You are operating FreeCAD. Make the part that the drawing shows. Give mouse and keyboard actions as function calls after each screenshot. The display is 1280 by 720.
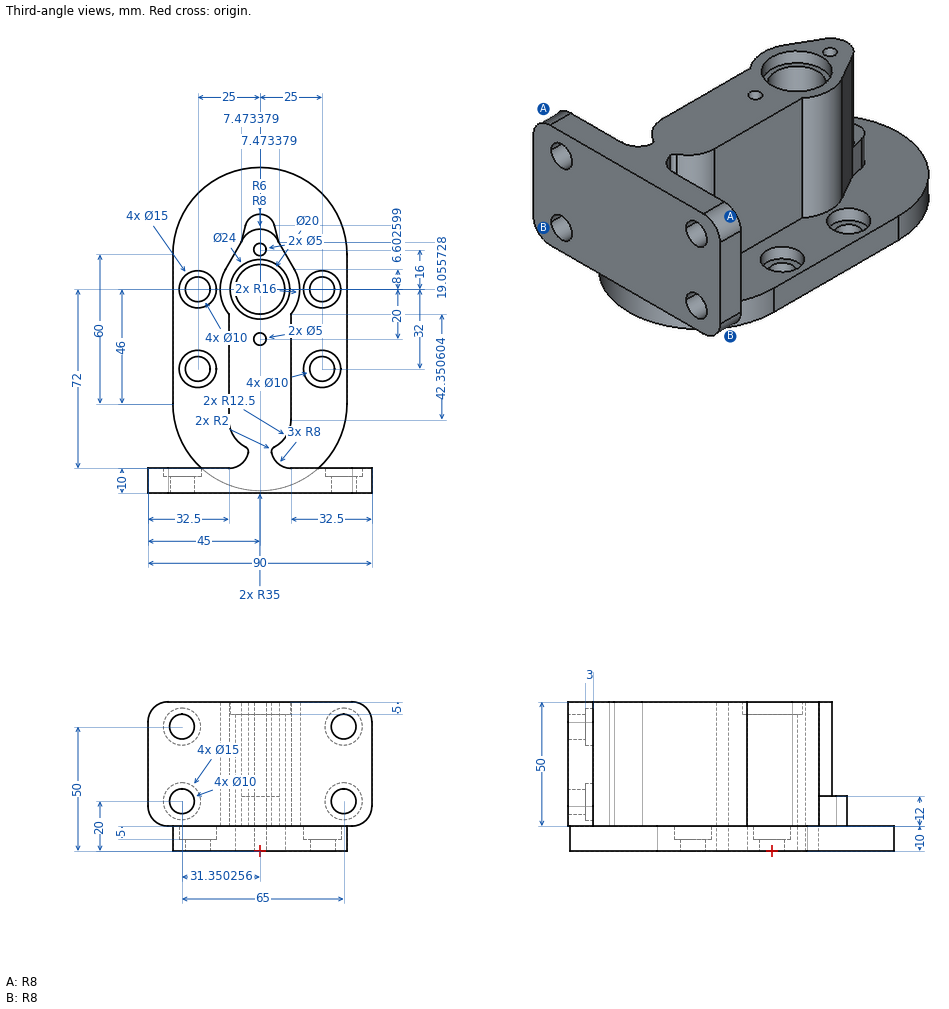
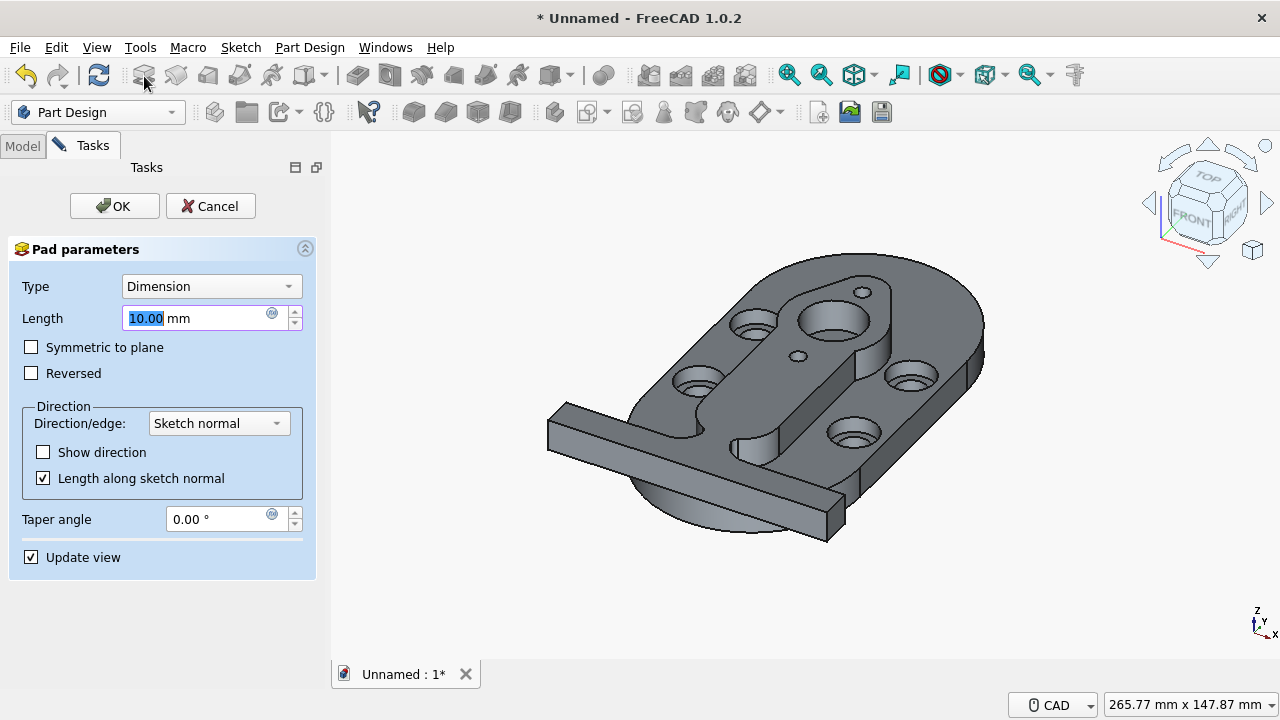
text(50)
key(Tab)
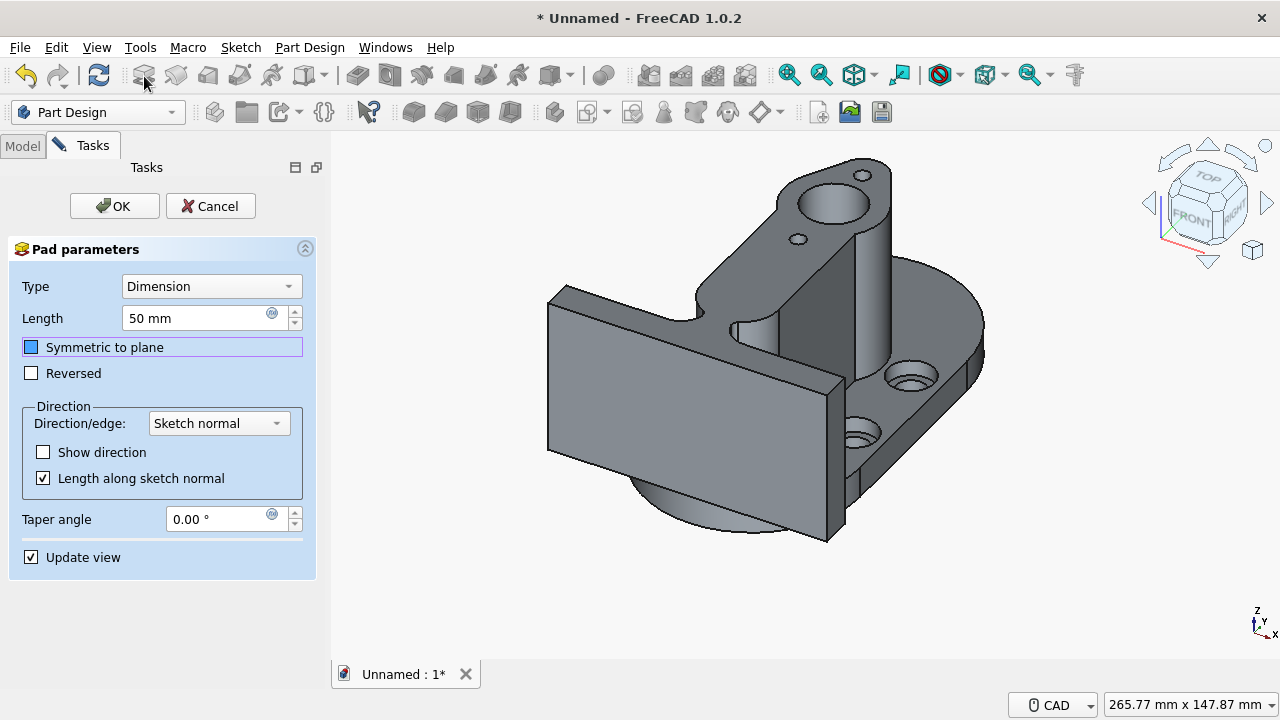
click(115, 206)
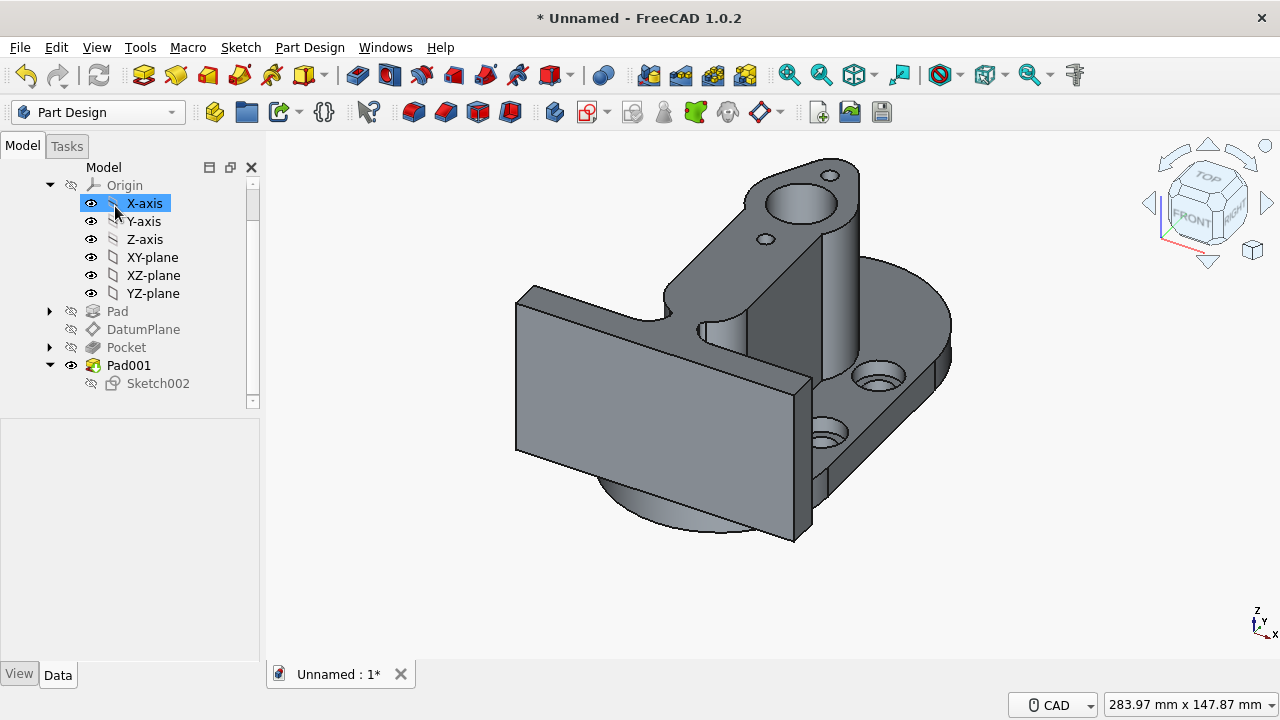
click(790, 76)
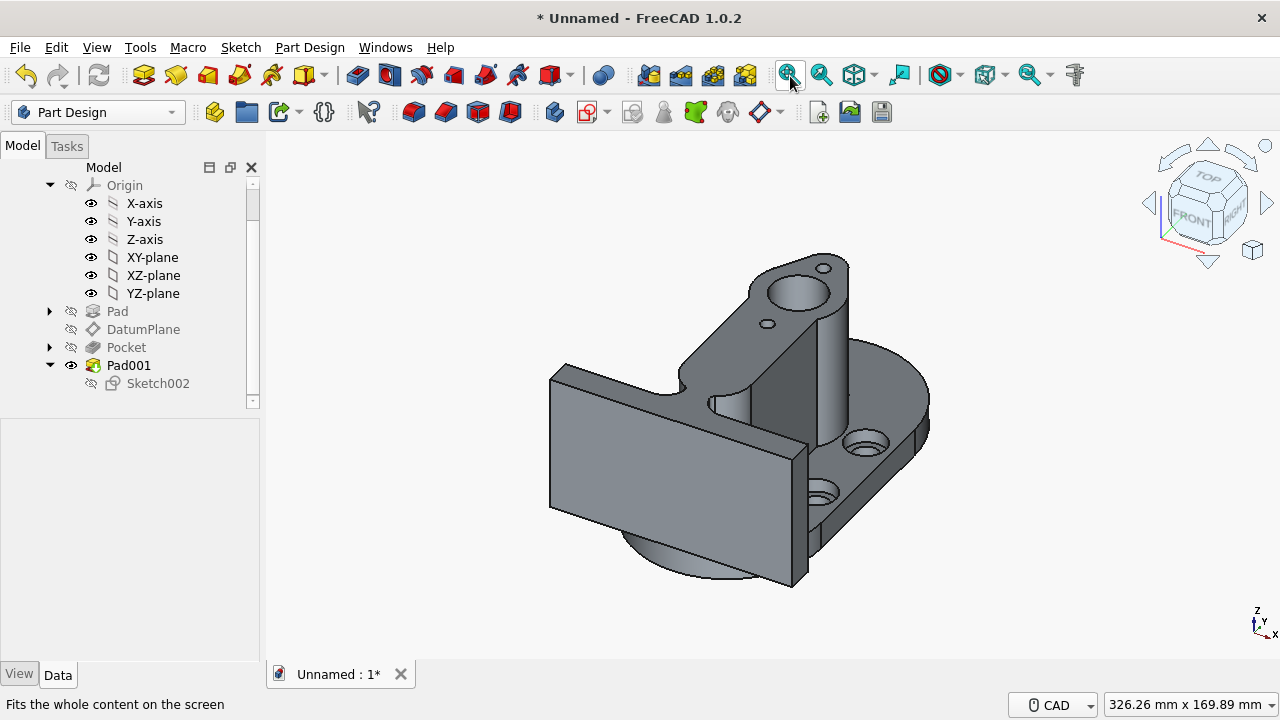
click(136, 257)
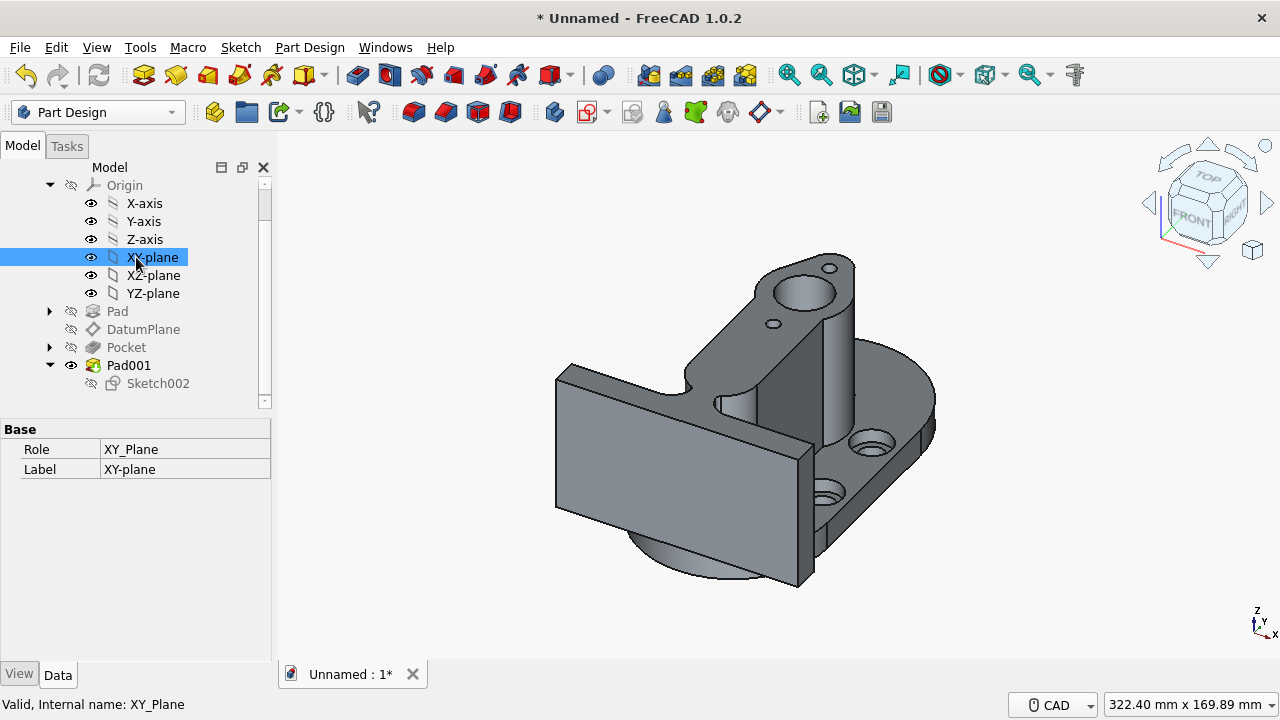
click(760, 112)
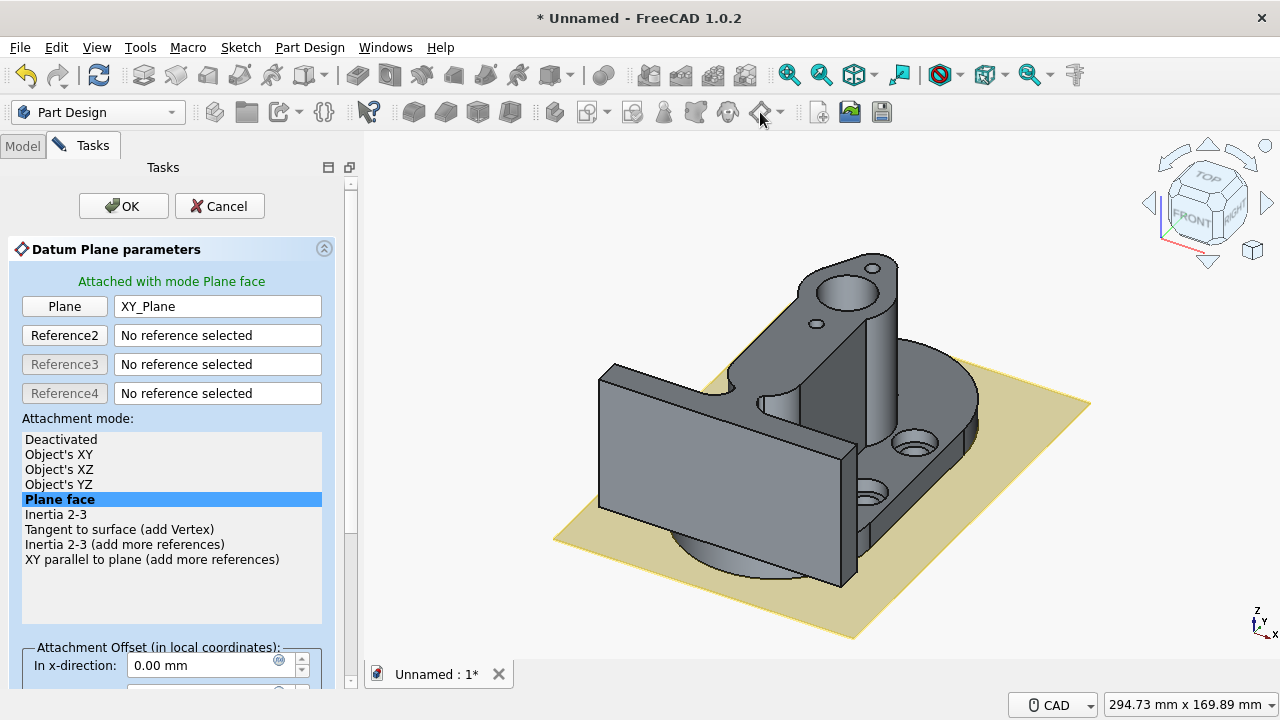
scroll(351, 432, down, 2)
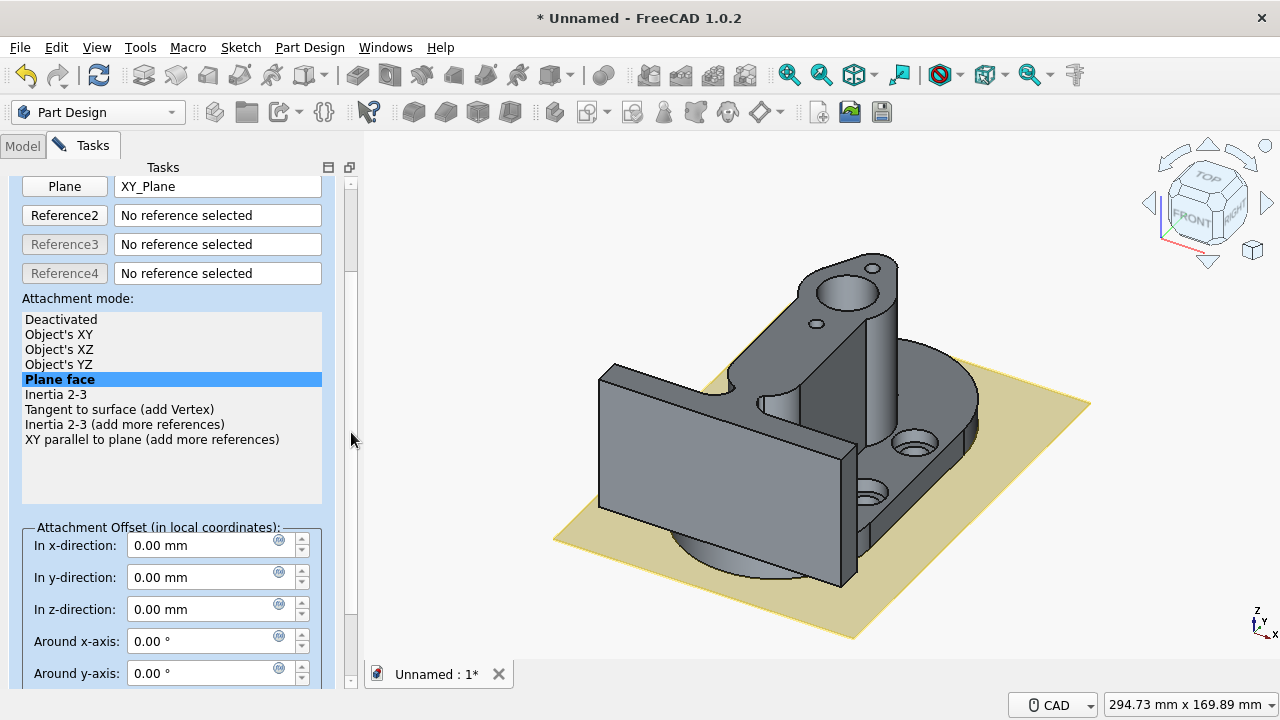
triple_click(210, 609)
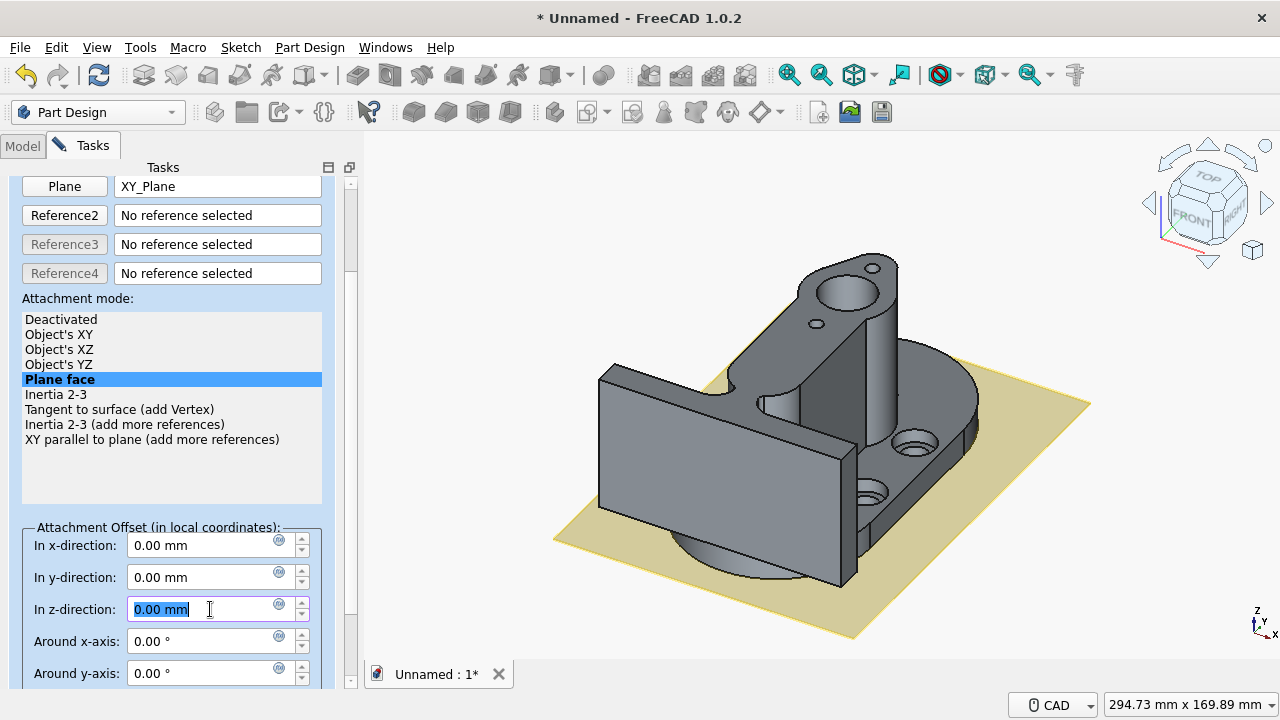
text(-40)
key(Tab)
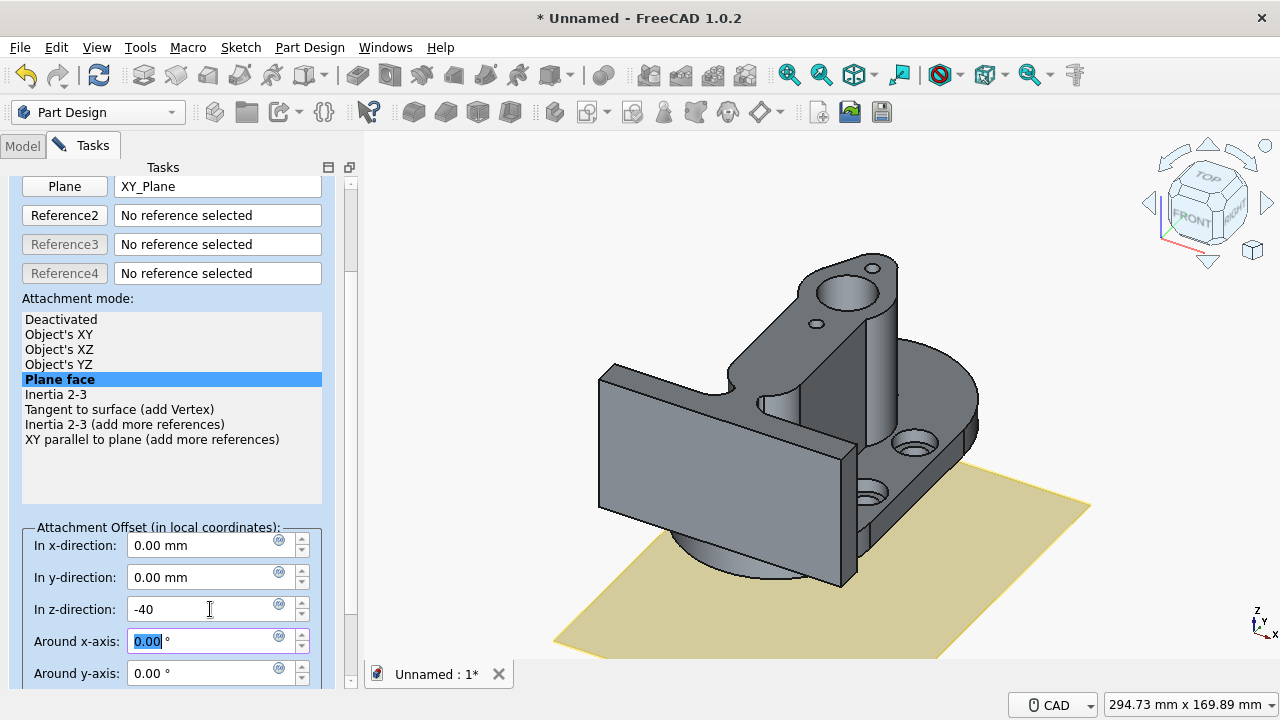
scroll(351, 432, up, 3)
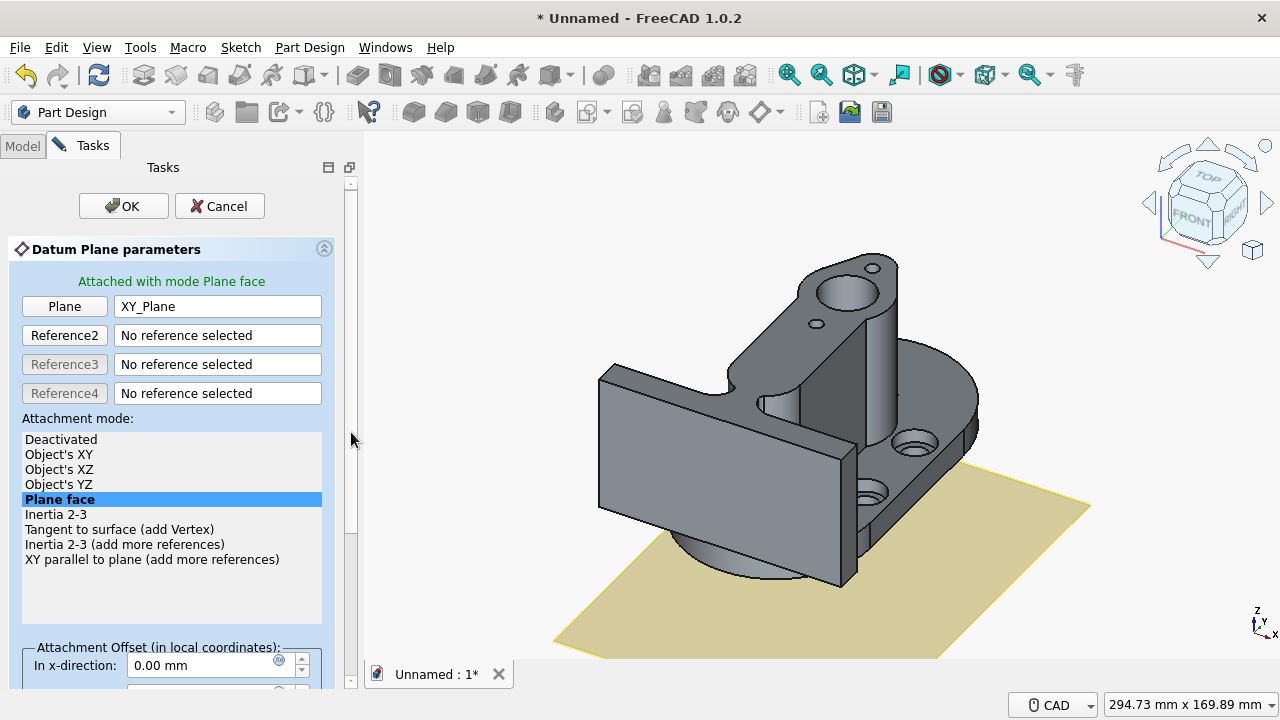
click(124, 206)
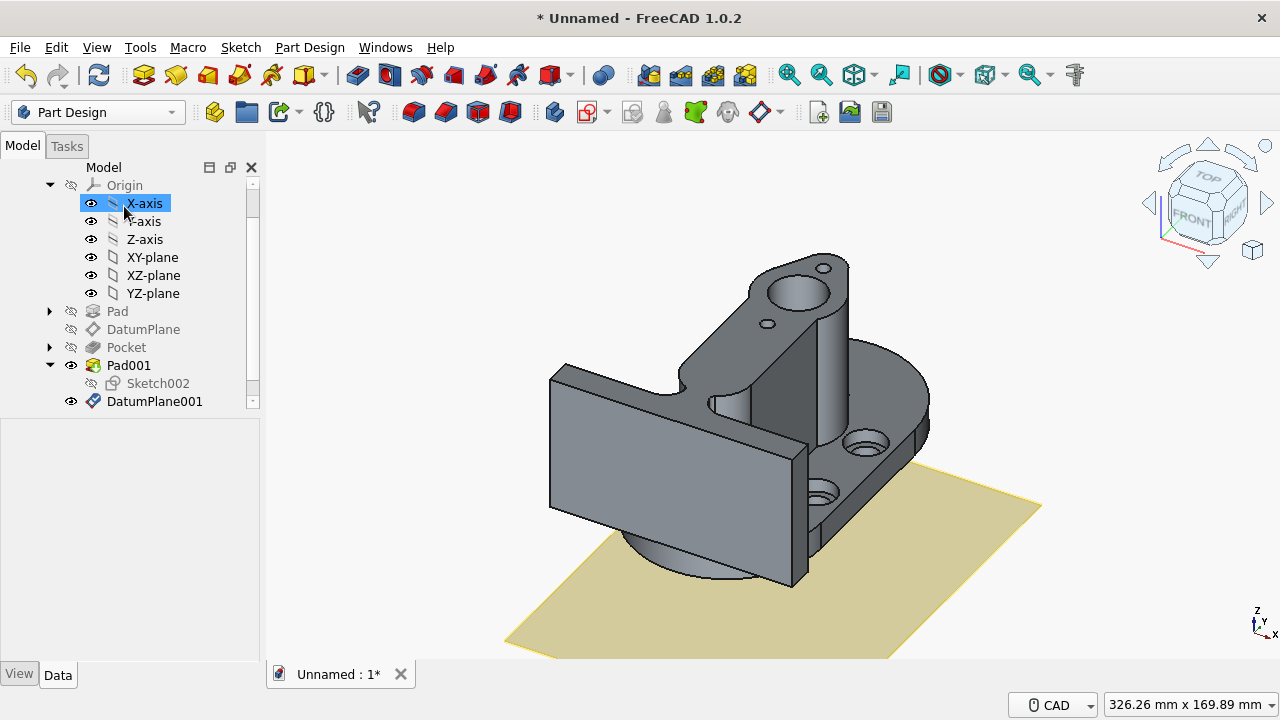
click(116, 401)